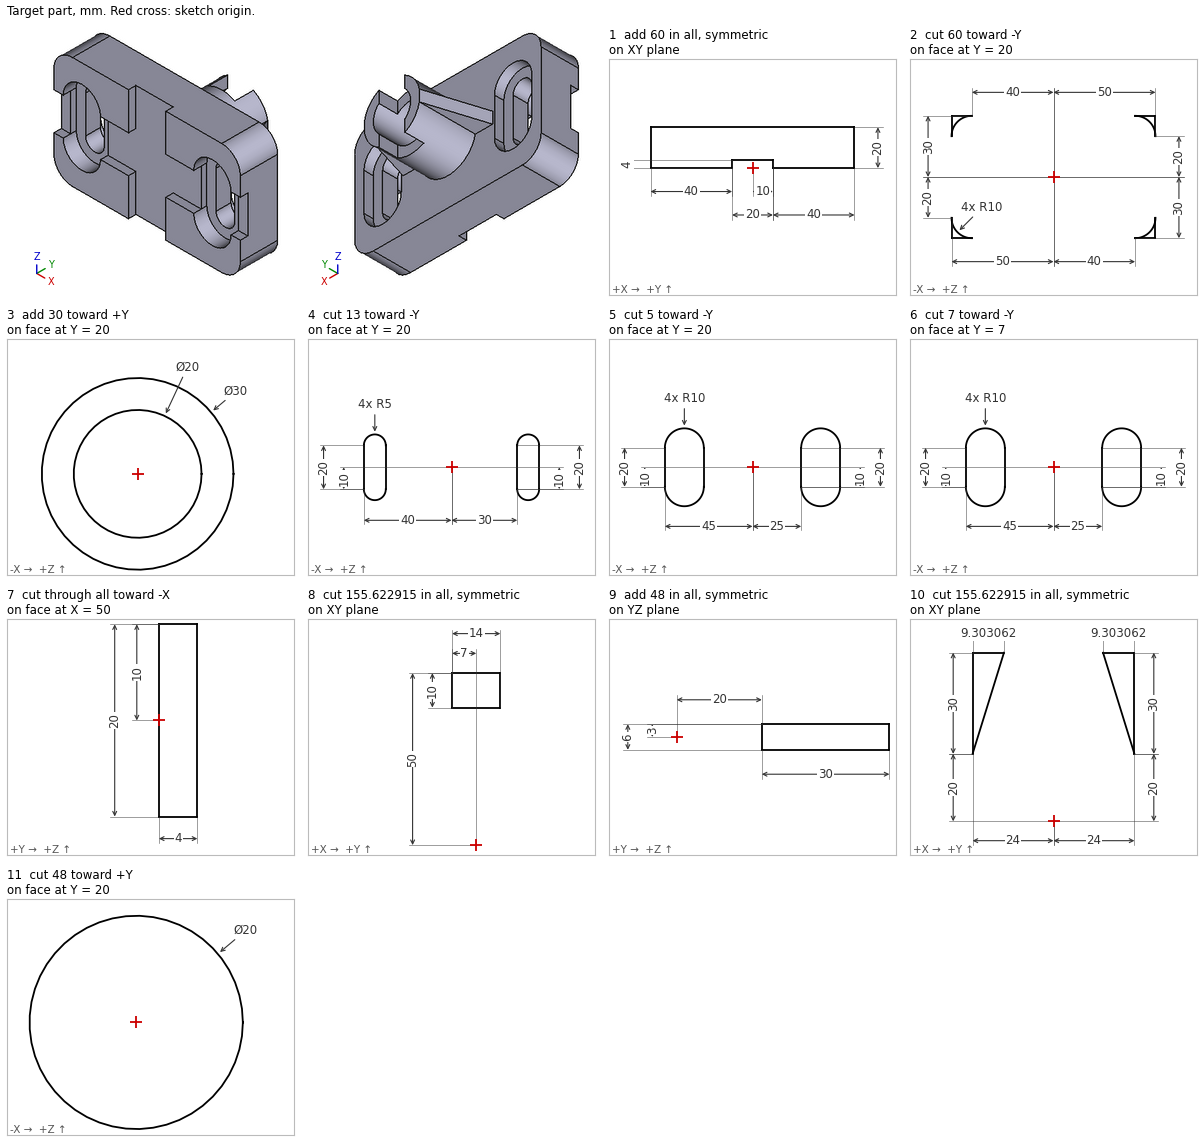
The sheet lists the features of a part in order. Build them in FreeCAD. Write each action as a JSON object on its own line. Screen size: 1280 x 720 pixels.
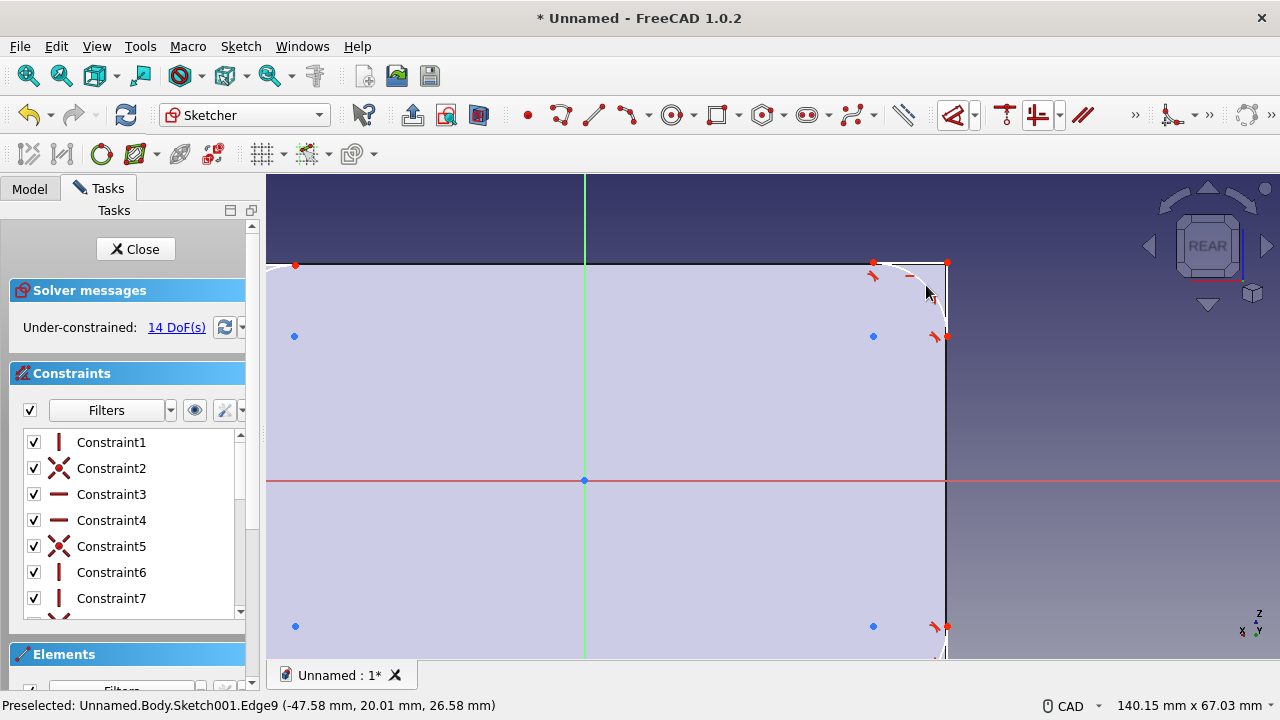
{"action": "scroll", "coordinate": [948, 286], "scroll_direction": "down", "scroll_amount": 2}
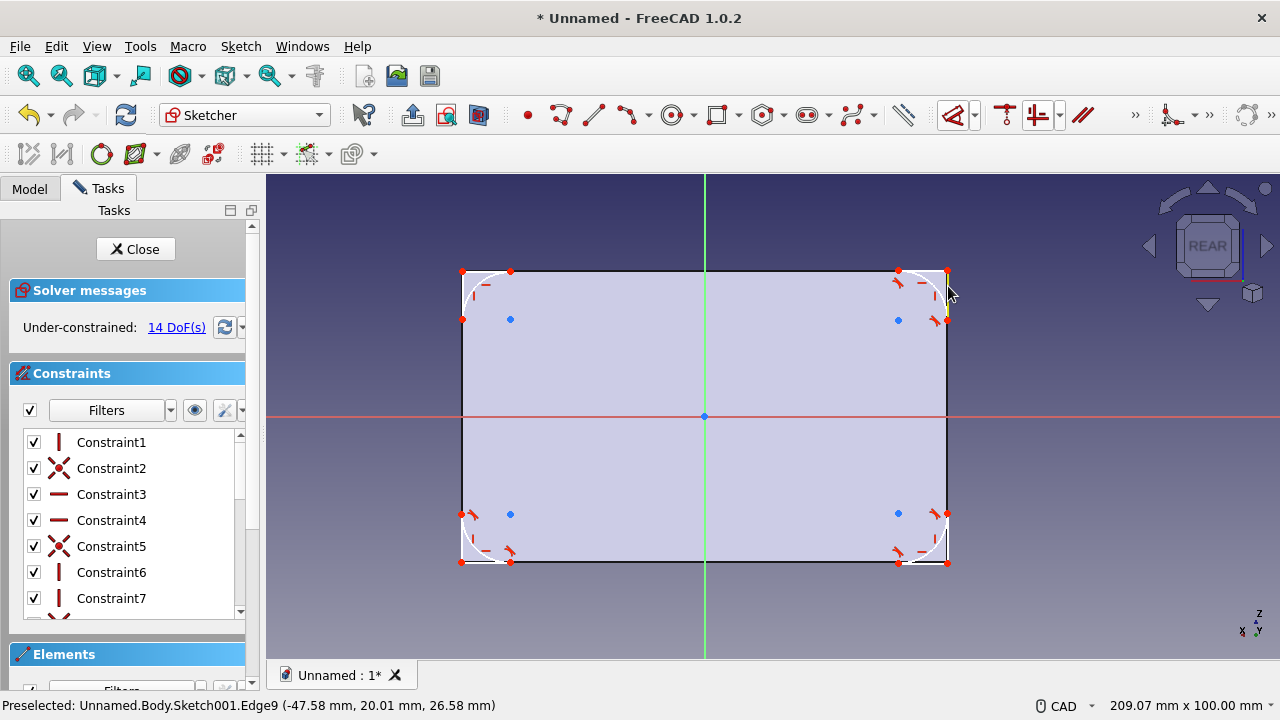
{"action": "scroll", "coordinate": [477, 272], "scroll_direction": "up", "scroll_amount": 2}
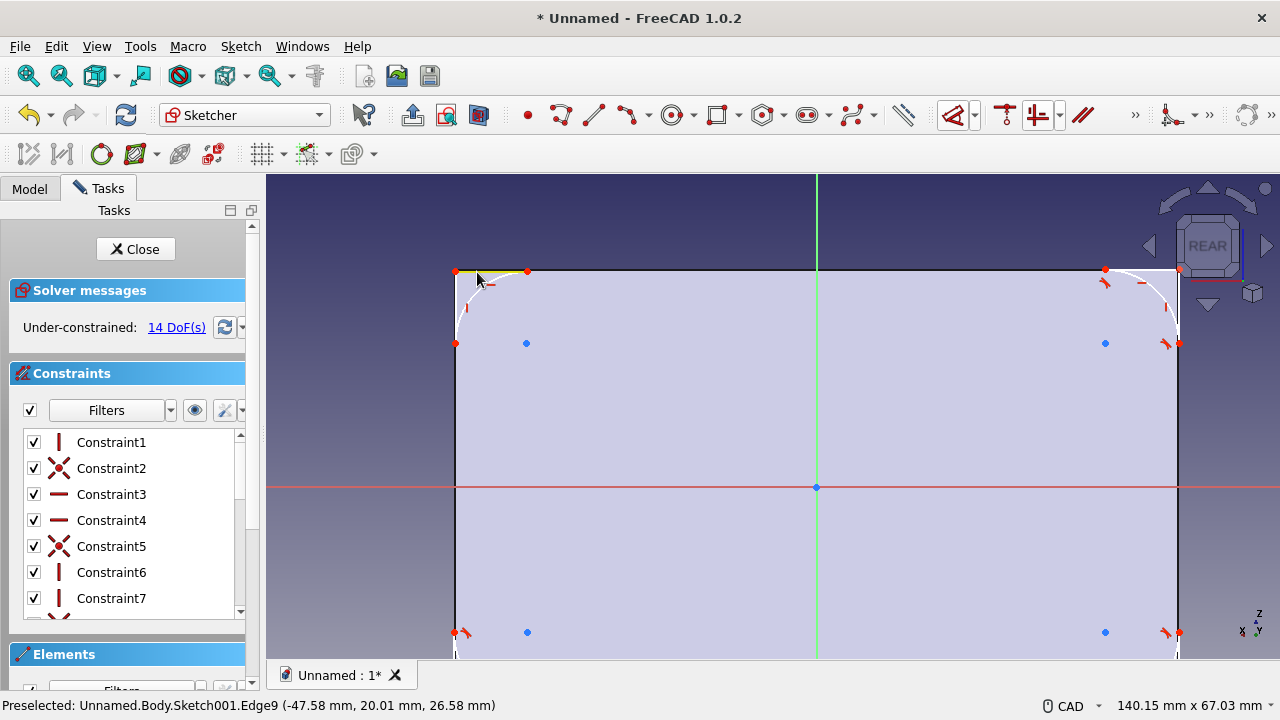
{"action": "left_click", "coordinate": [477, 272]}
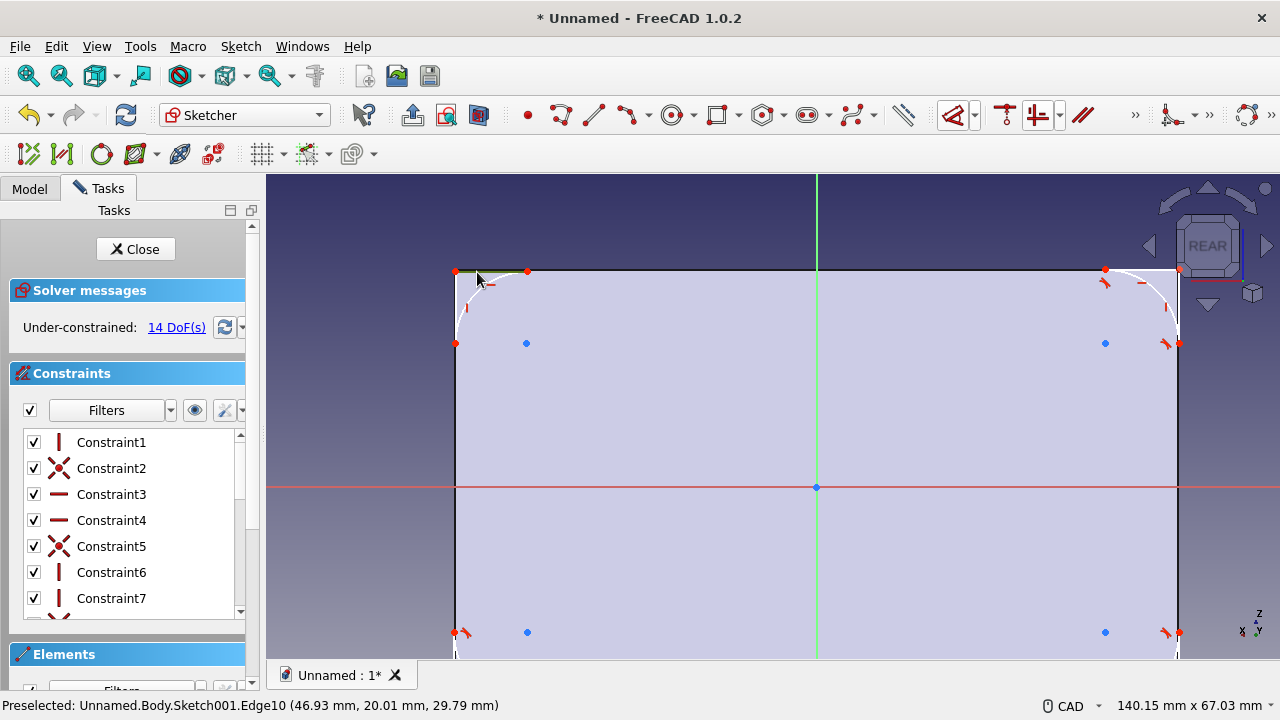
{"action": "left_click", "coordinate": [476, 293]}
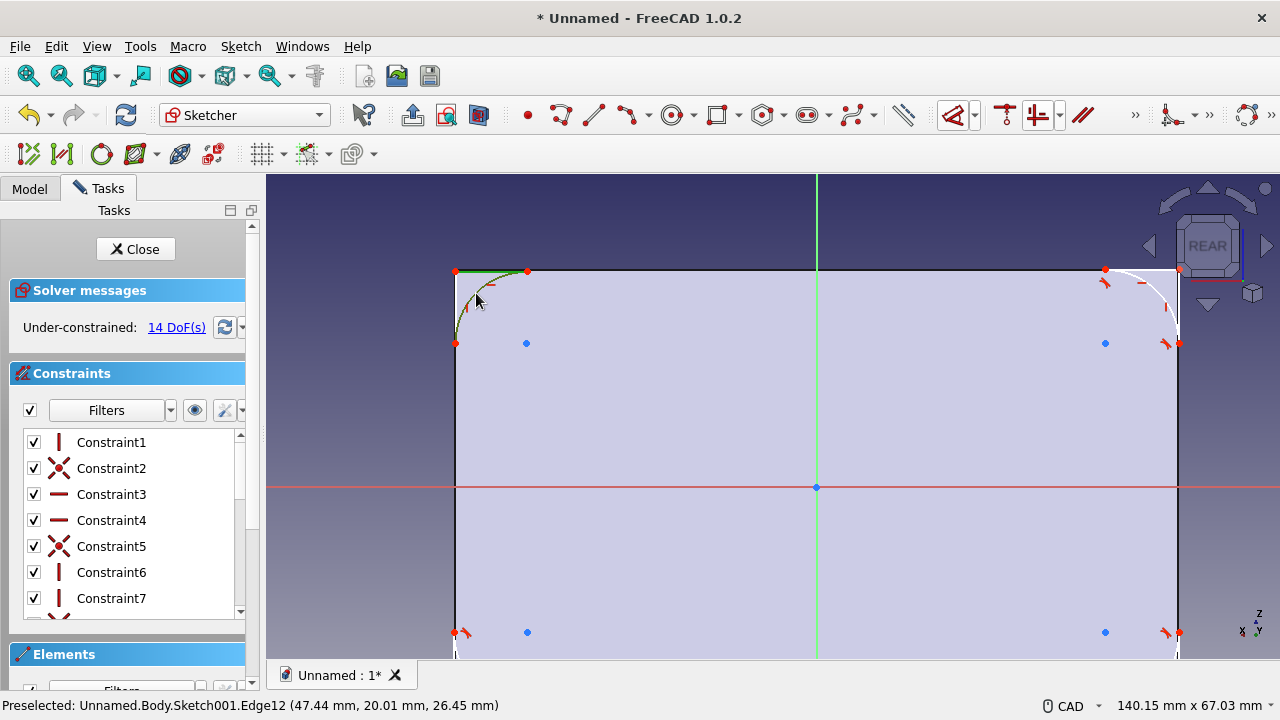
{"action": "key", "text": "t"}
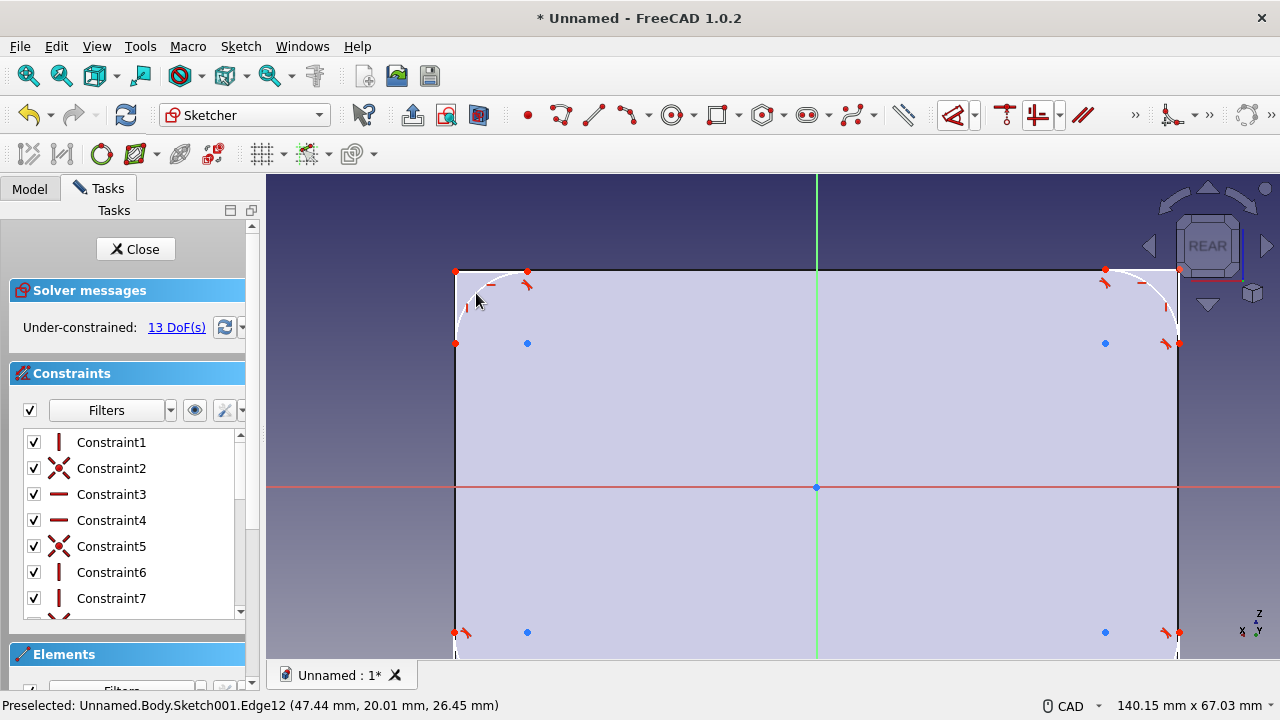
{"action": "left_click", "coordinate": [456, 293]}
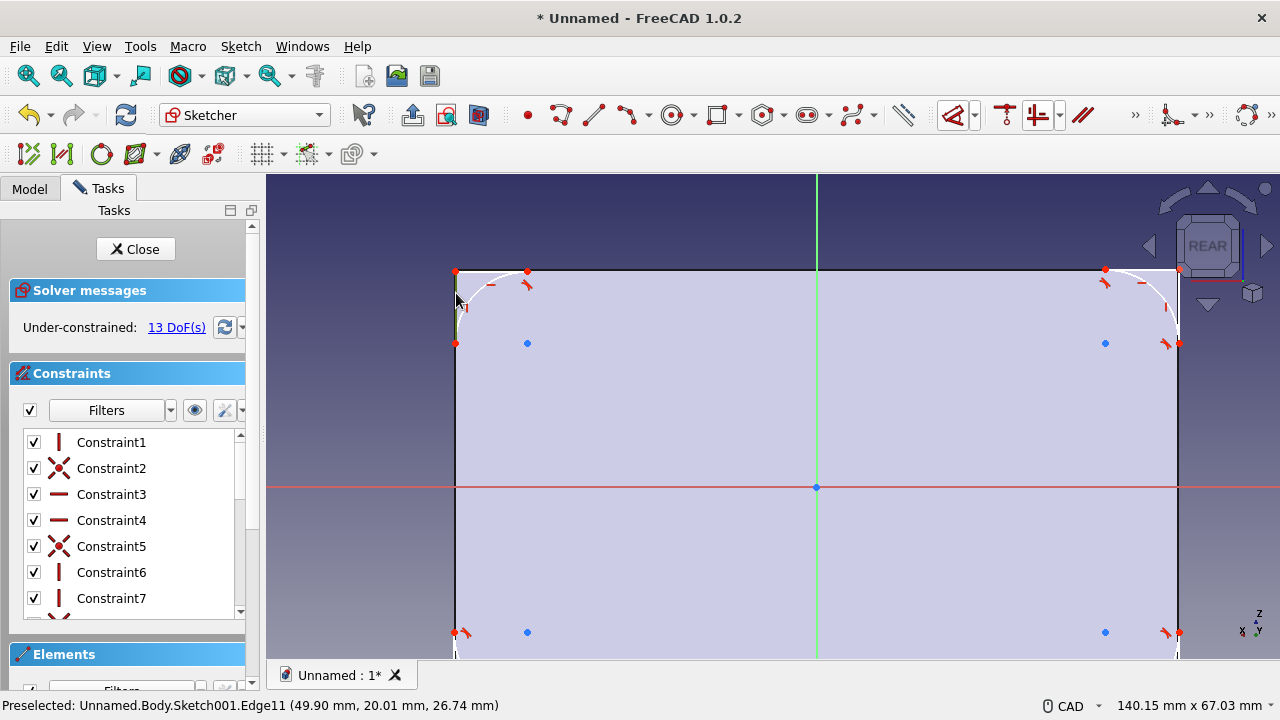
{"action": "left_click", "coordinate": [477, 293]}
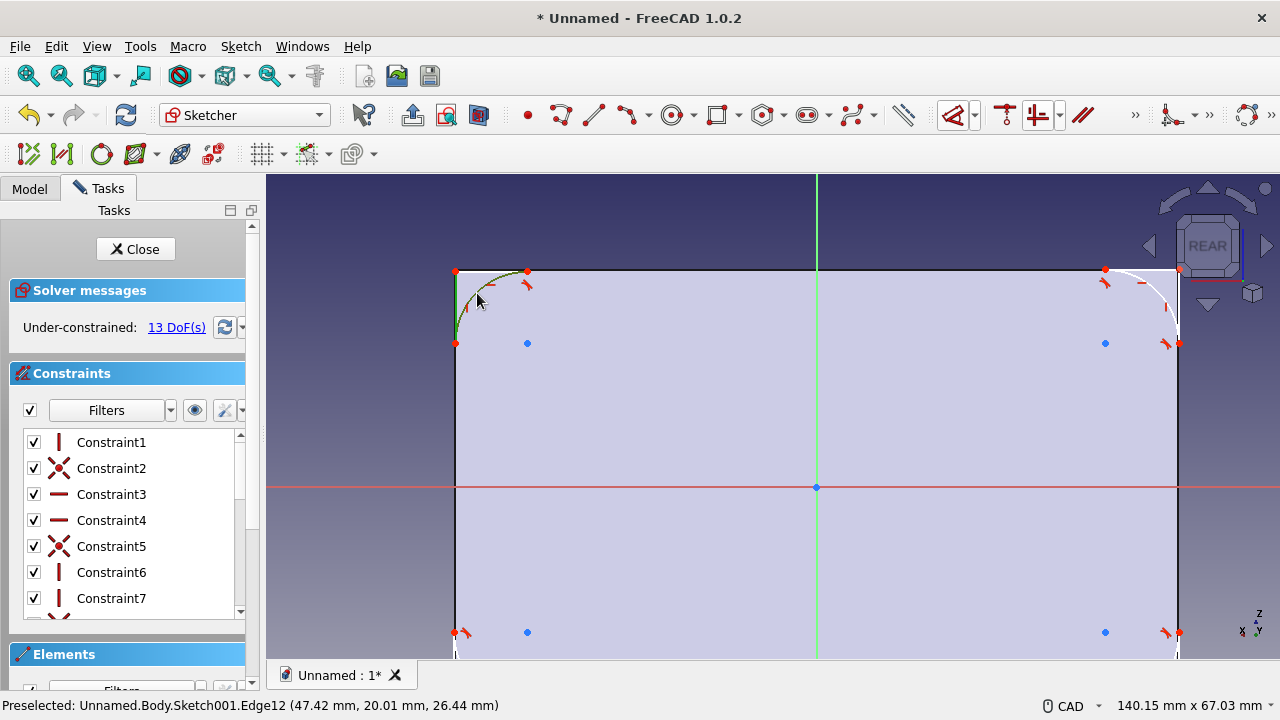
{"action": "key", "text": "t"}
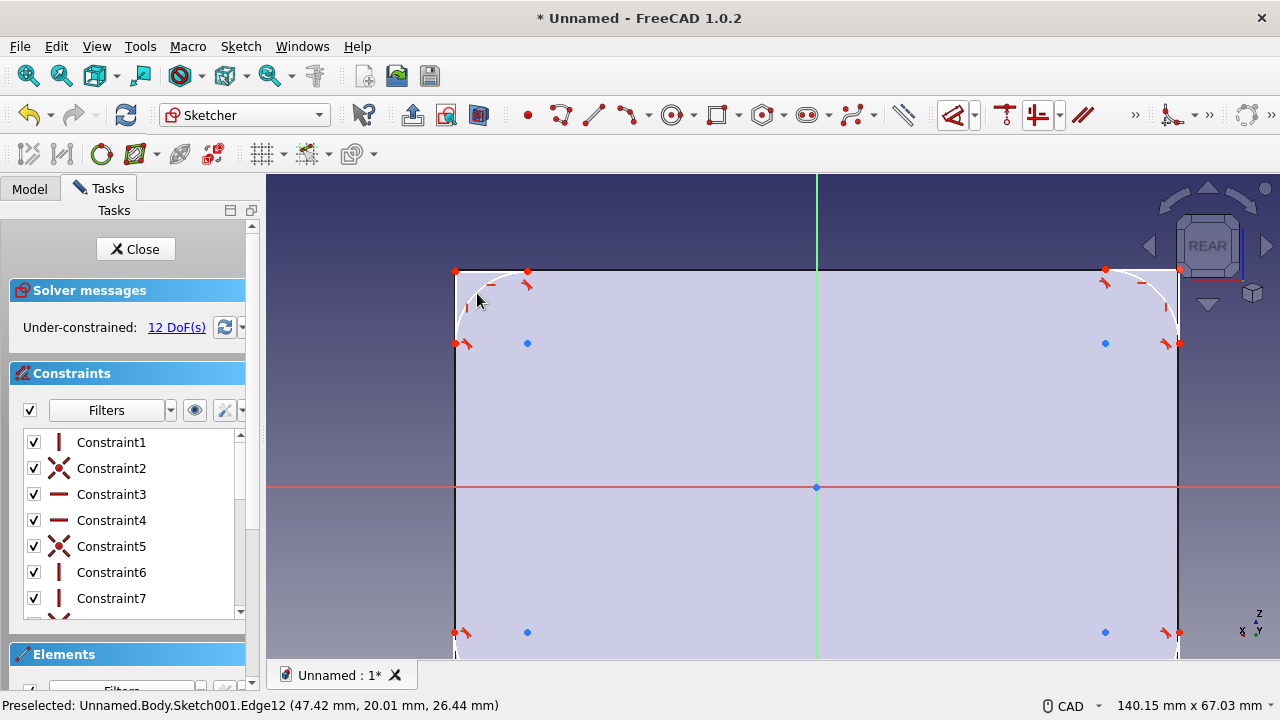
{"action": "scroll", "coordinate": [477, 272], "scroll_direction": "down", "scroll_amount": 2}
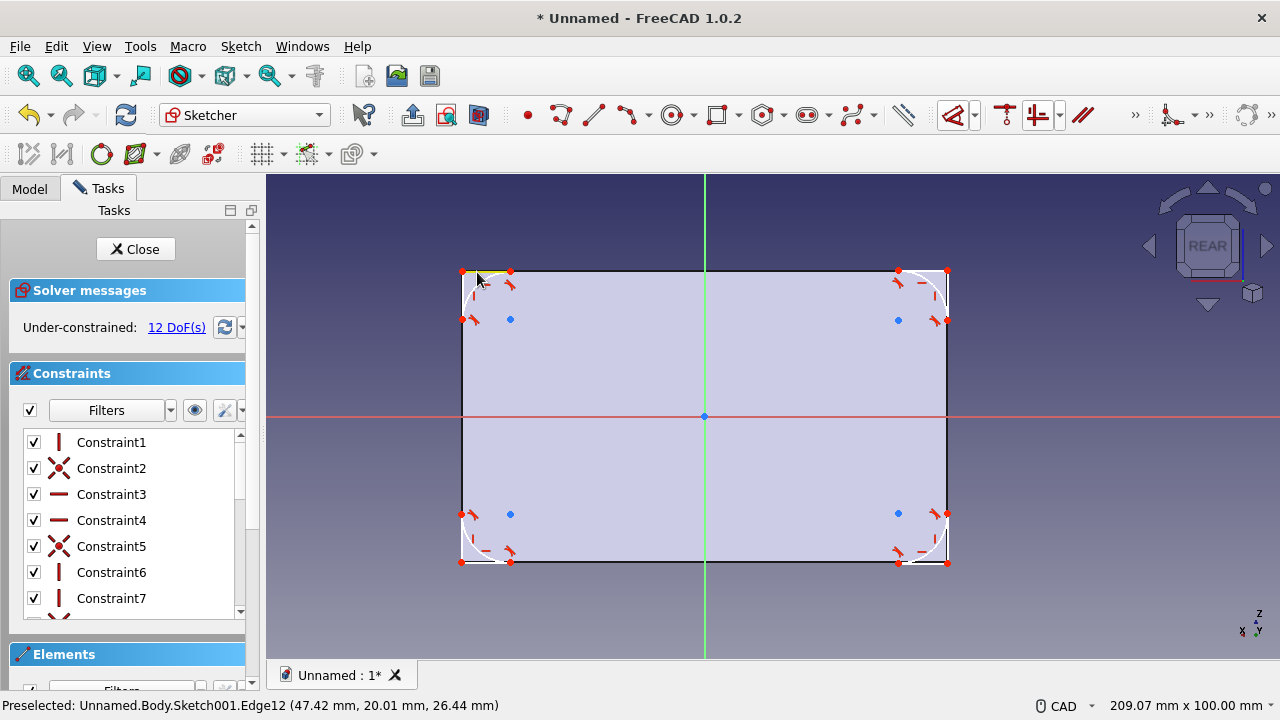
{"action": "left_click", "coordinate": [476, 549]}